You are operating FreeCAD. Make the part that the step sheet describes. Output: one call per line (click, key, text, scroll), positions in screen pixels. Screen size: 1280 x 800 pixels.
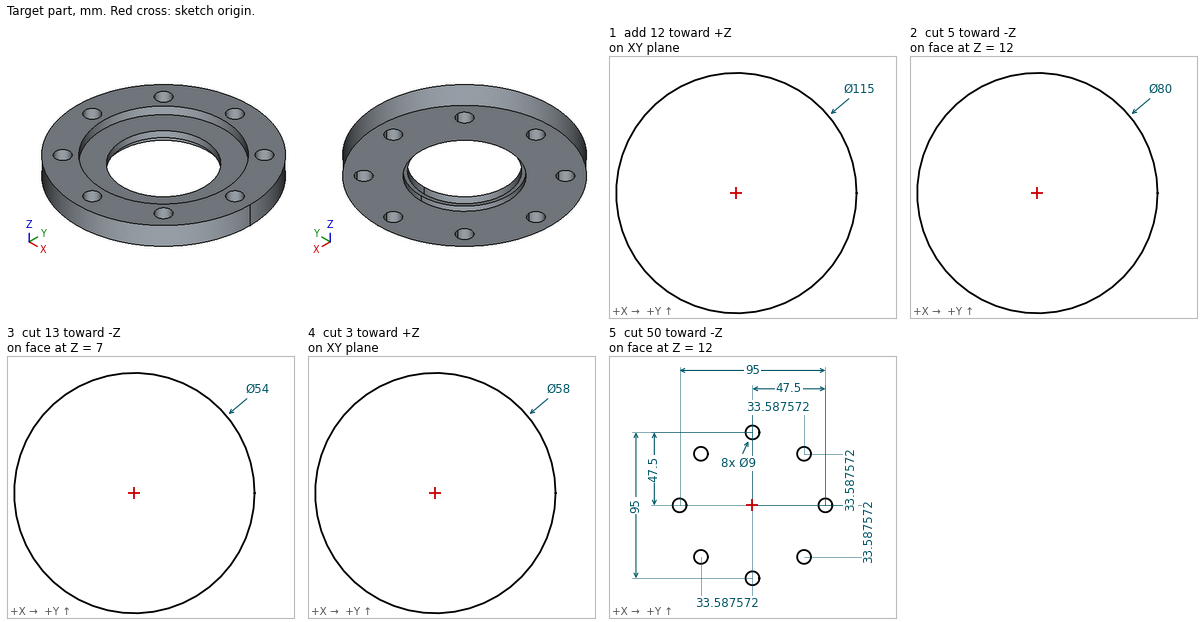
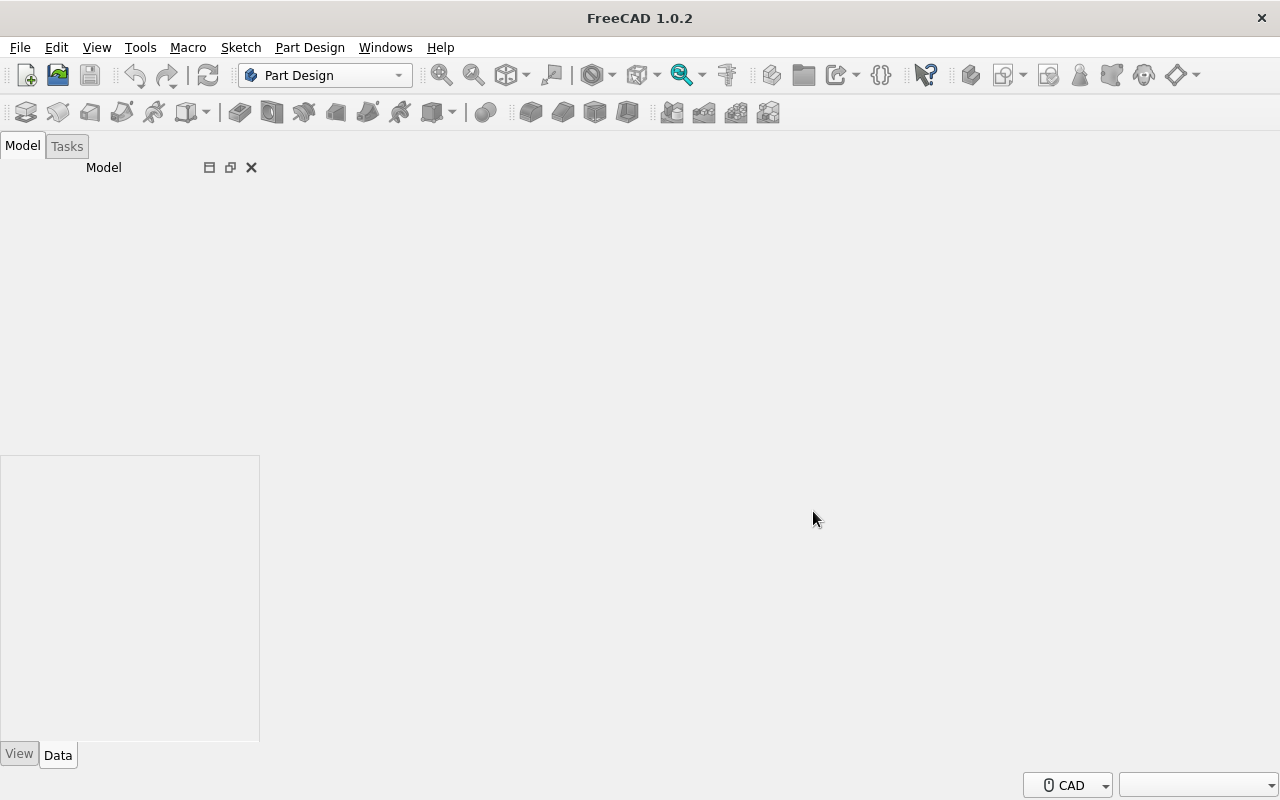
click(26, 76)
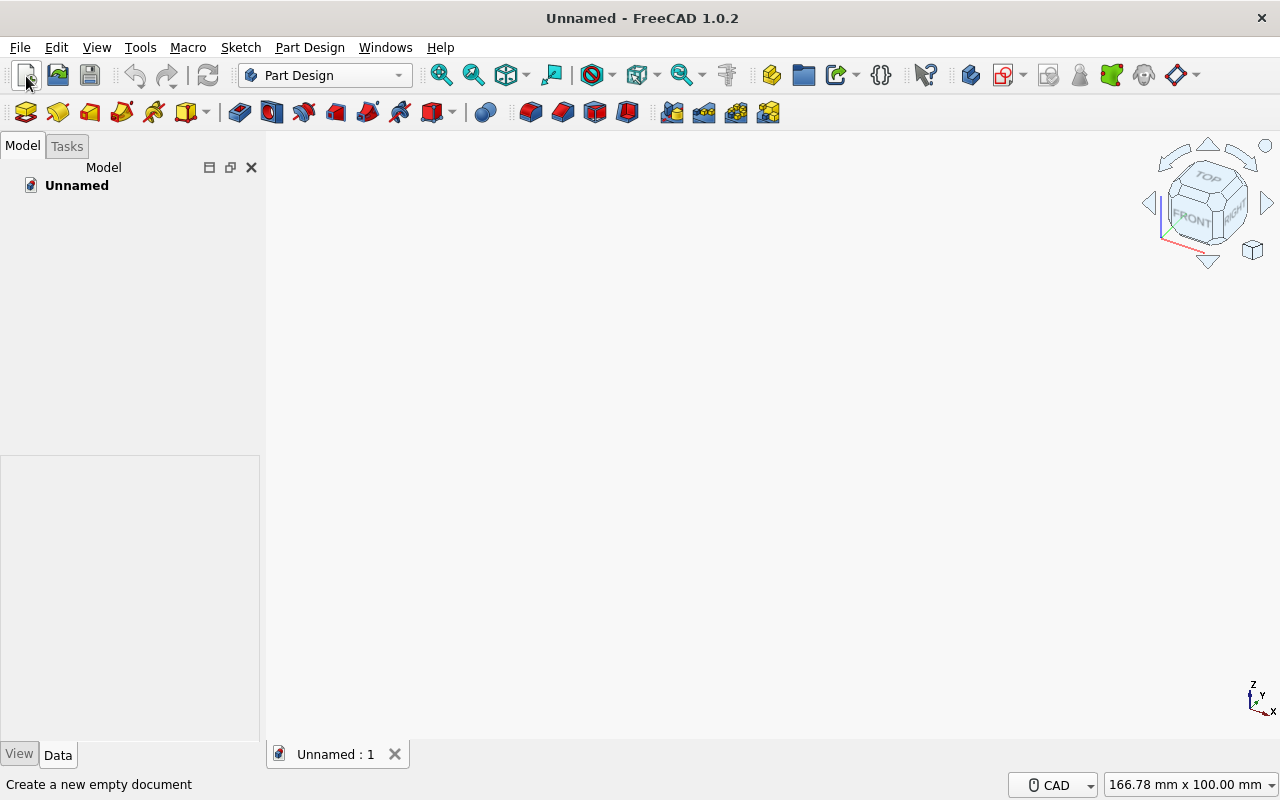
click(1004, 76)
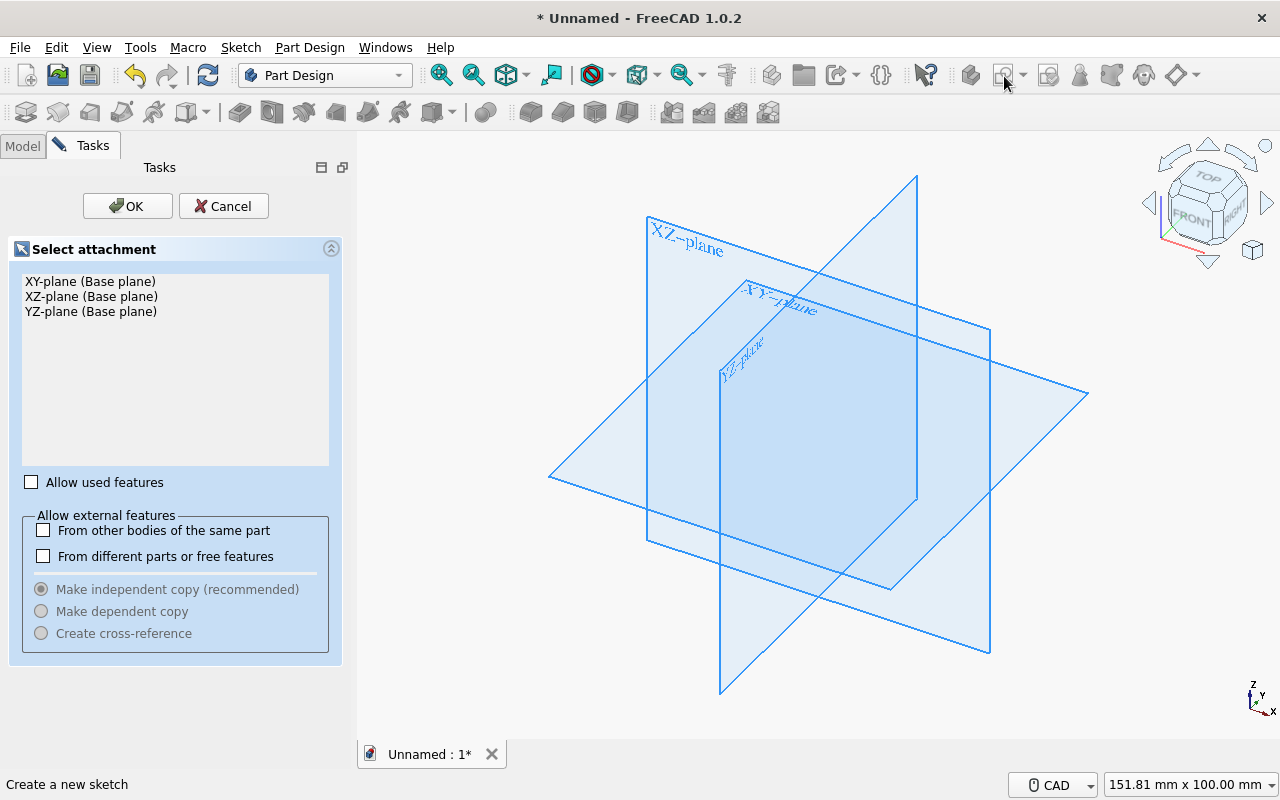
click(82, 282)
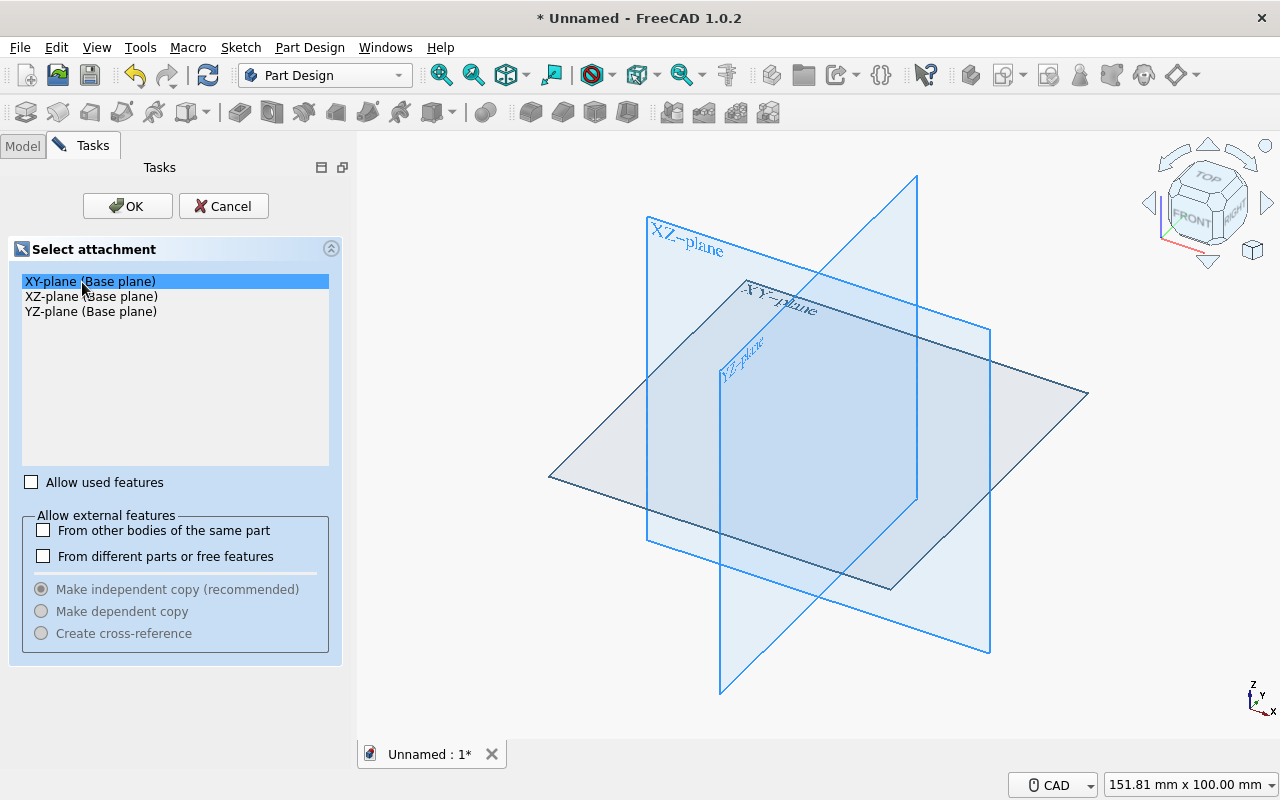
click(128, 206)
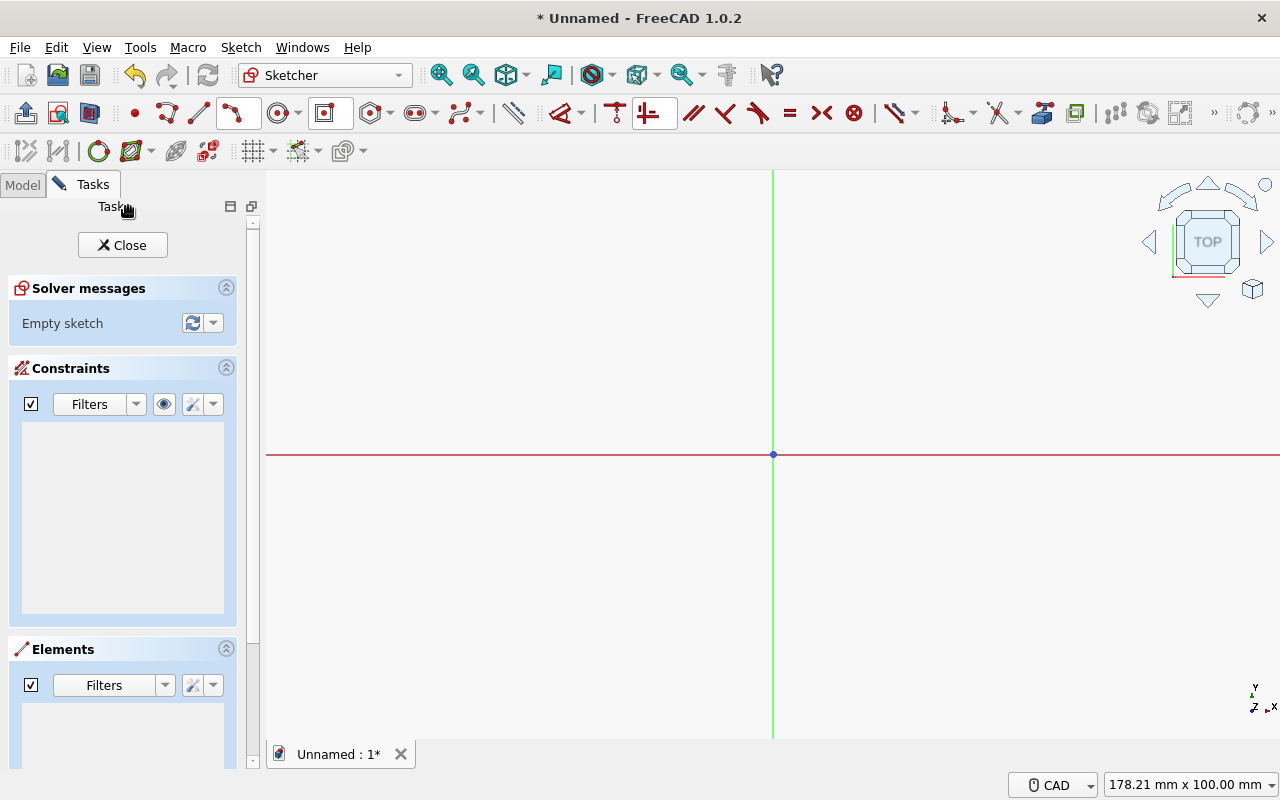
scroll(621, 454, down, 3)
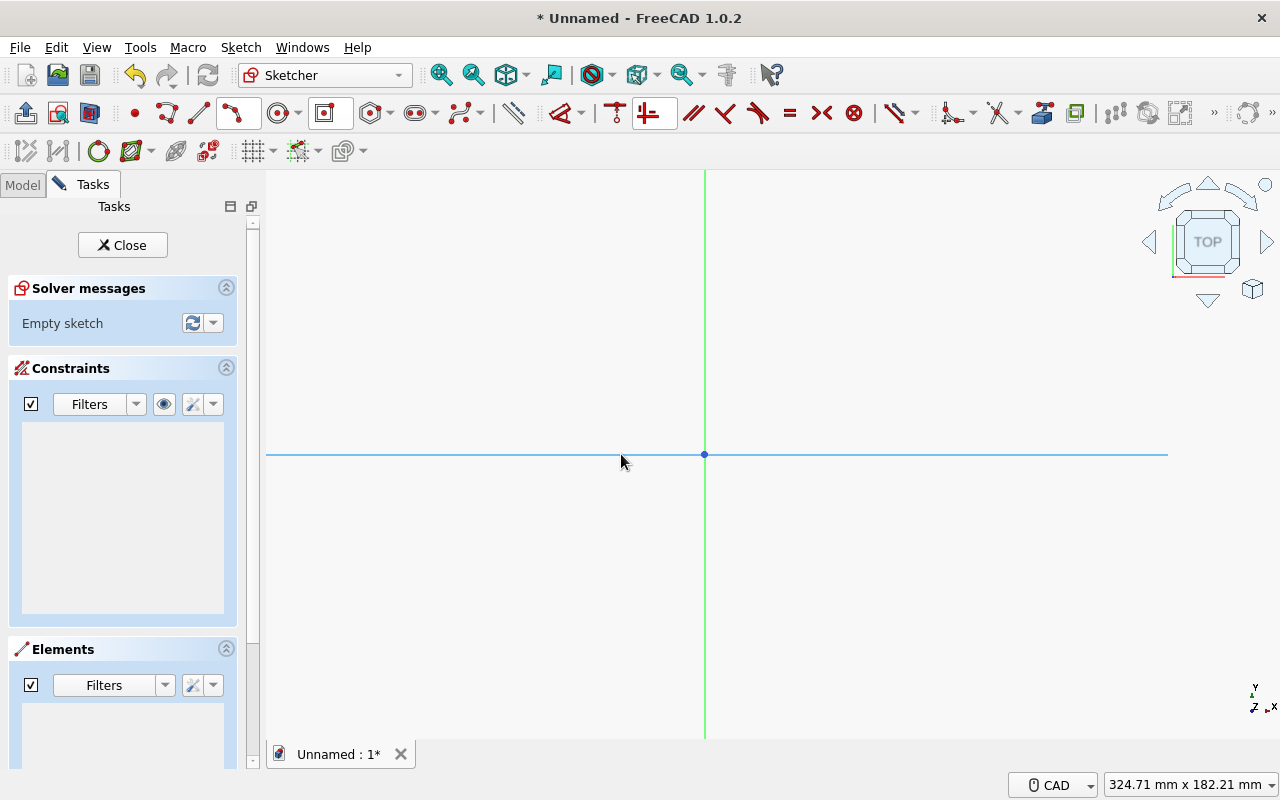
click(278, 114)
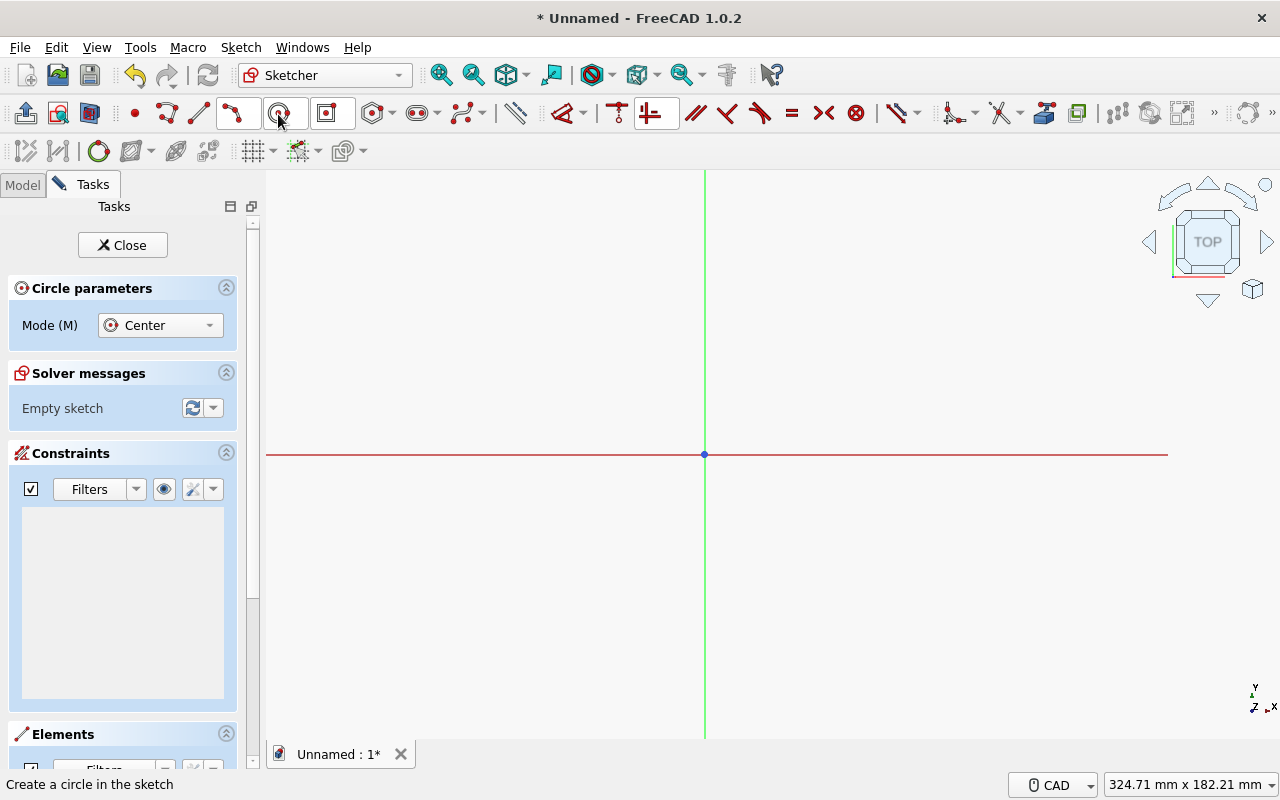
click(705, 454)
move(832, 328)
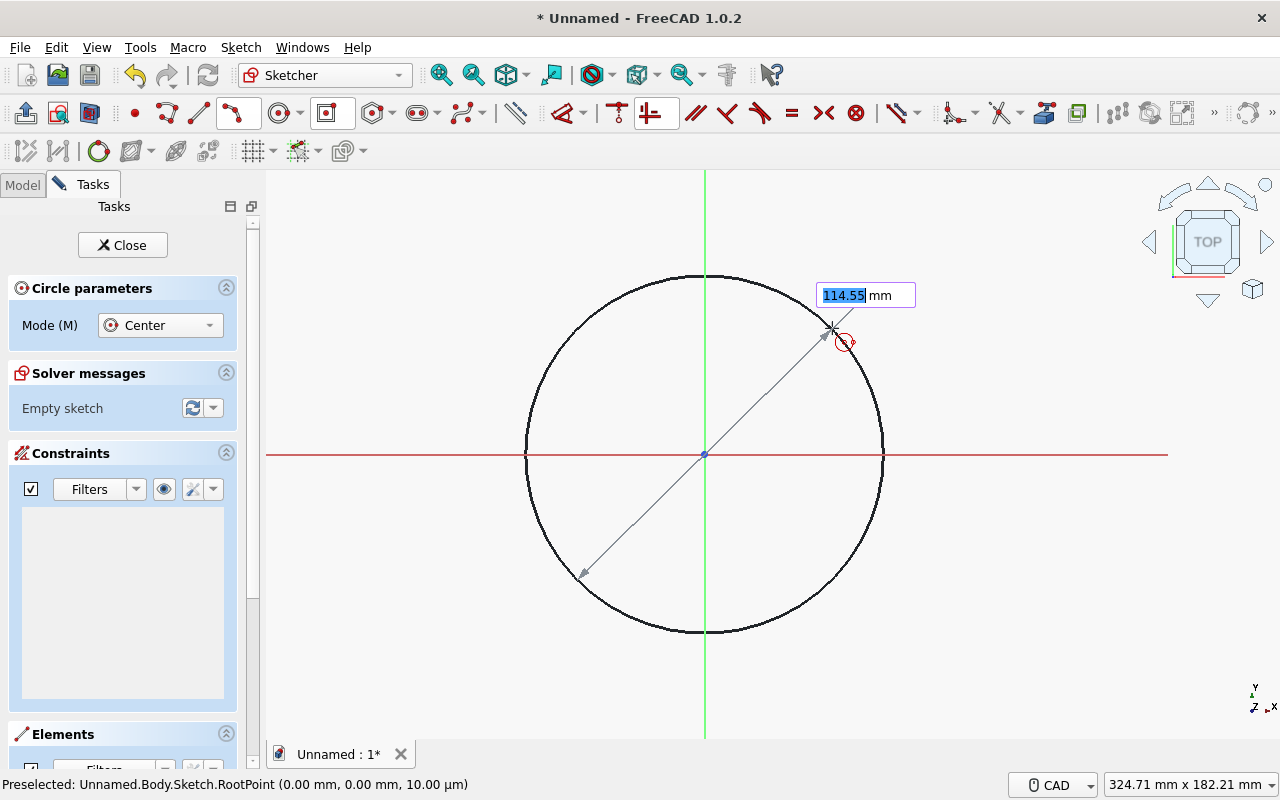
text(115)
key(Return)
key(Escape)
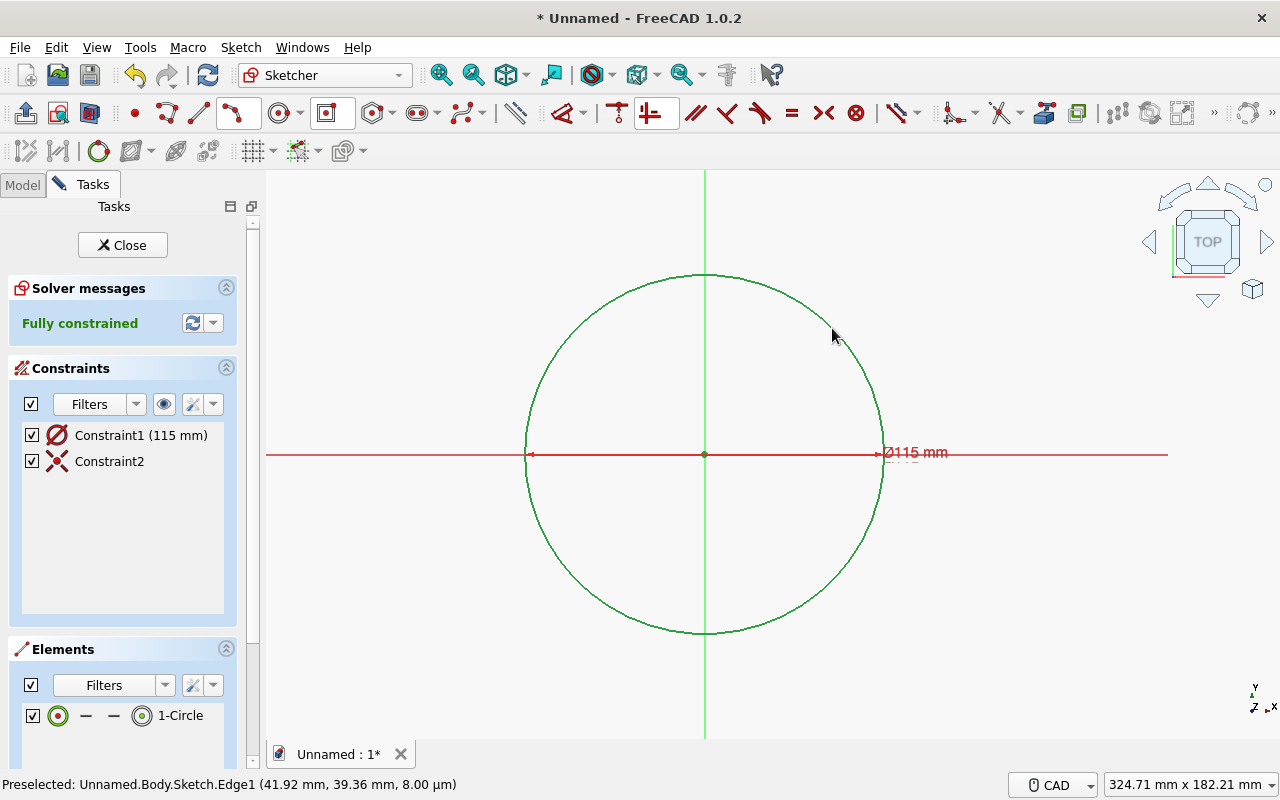
click(123, 245)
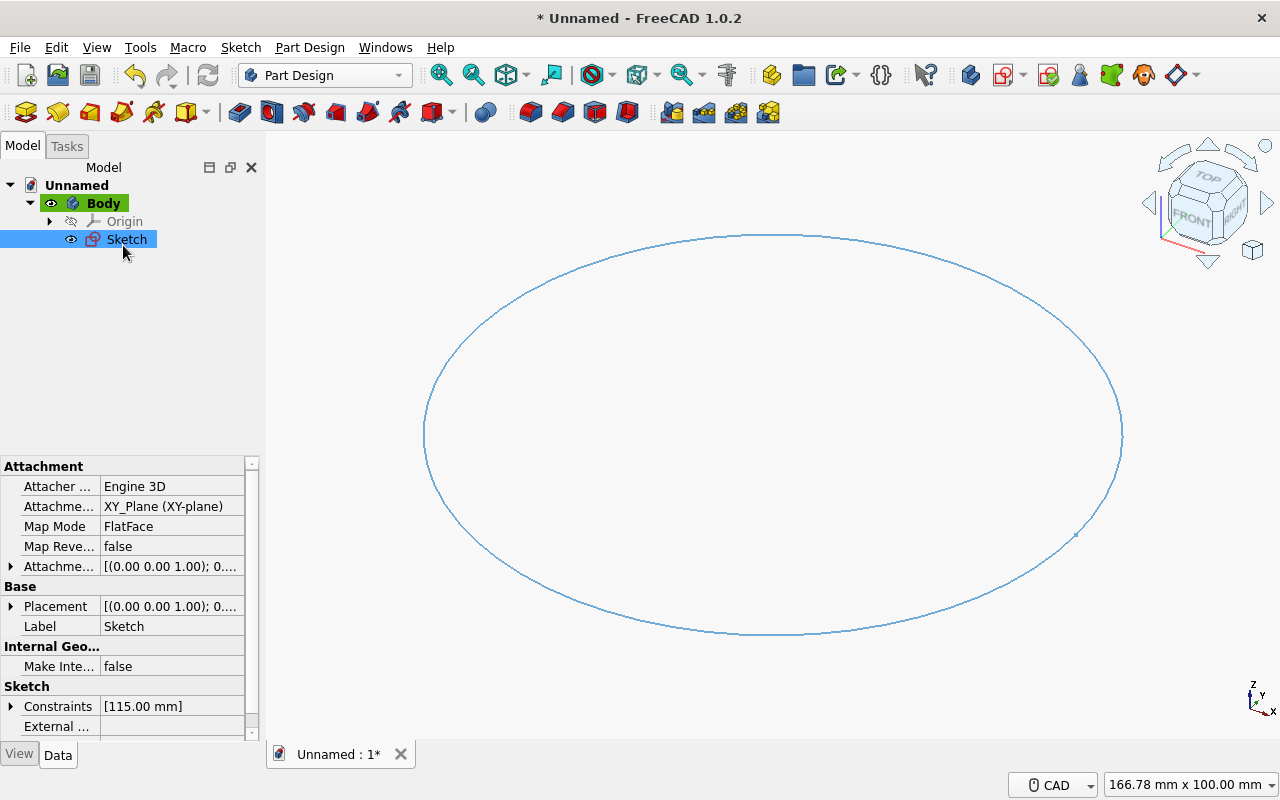
click(26, 112)